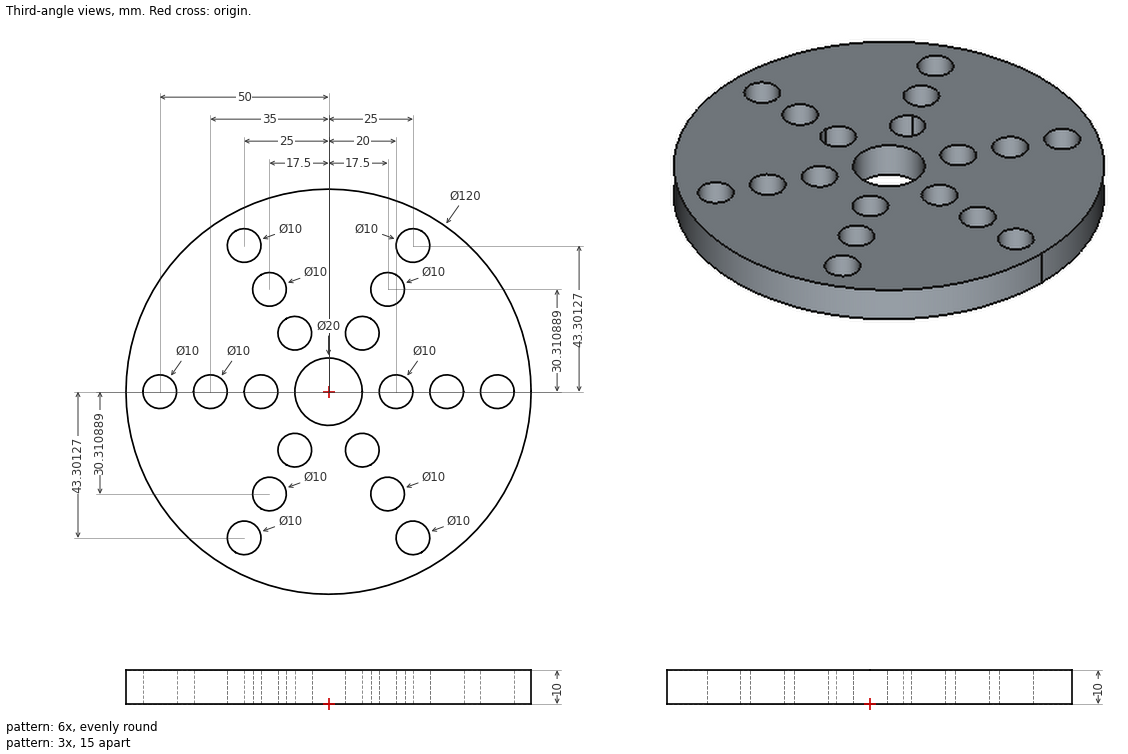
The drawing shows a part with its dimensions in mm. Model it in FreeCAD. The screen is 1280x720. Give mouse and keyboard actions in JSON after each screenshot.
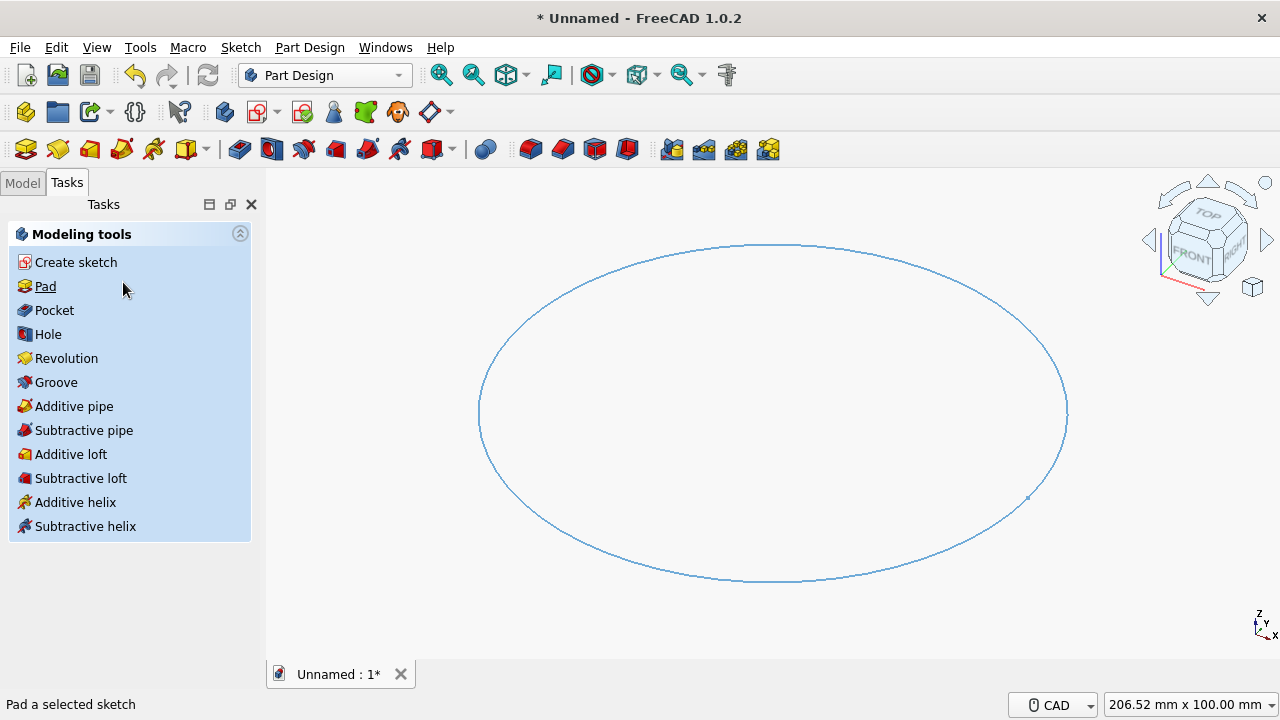
{"action": "left_click", "coordinate": [26, 150]}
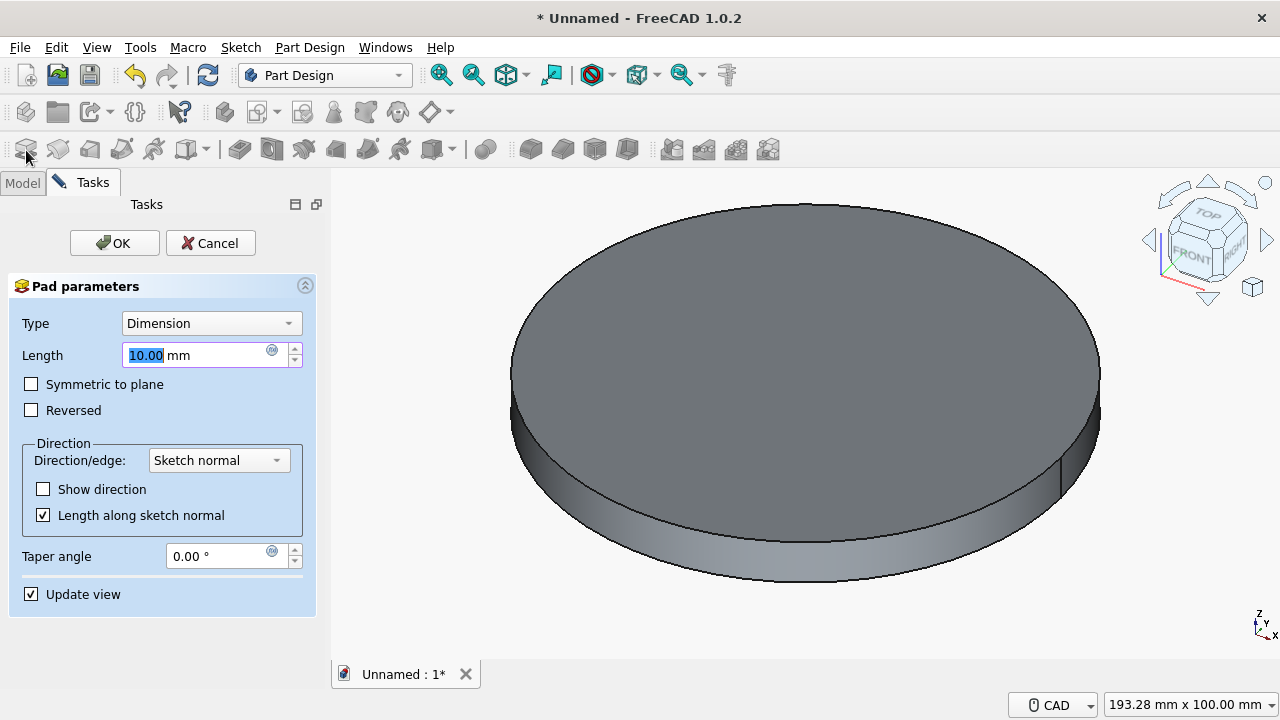
{"action": "type", "text": "10"}
{"action": "key", "text": "Tab"}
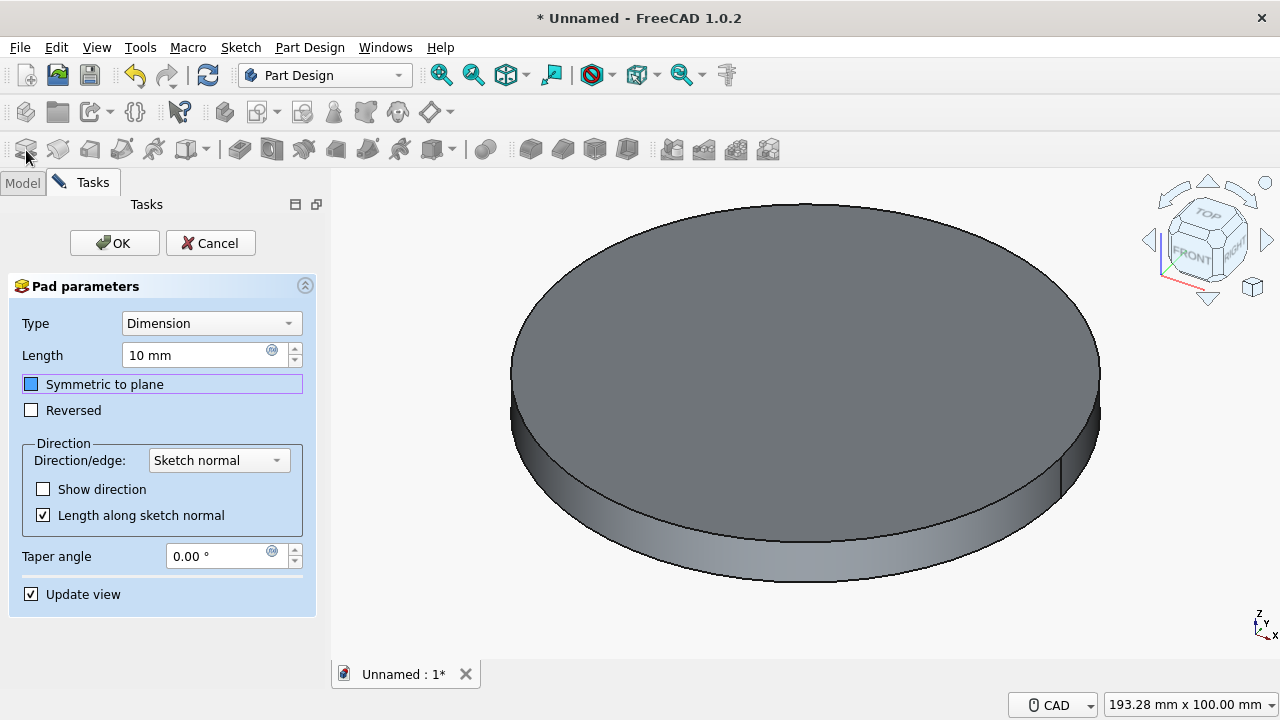
{"action": "left_click", "coordinate": [115, 243]}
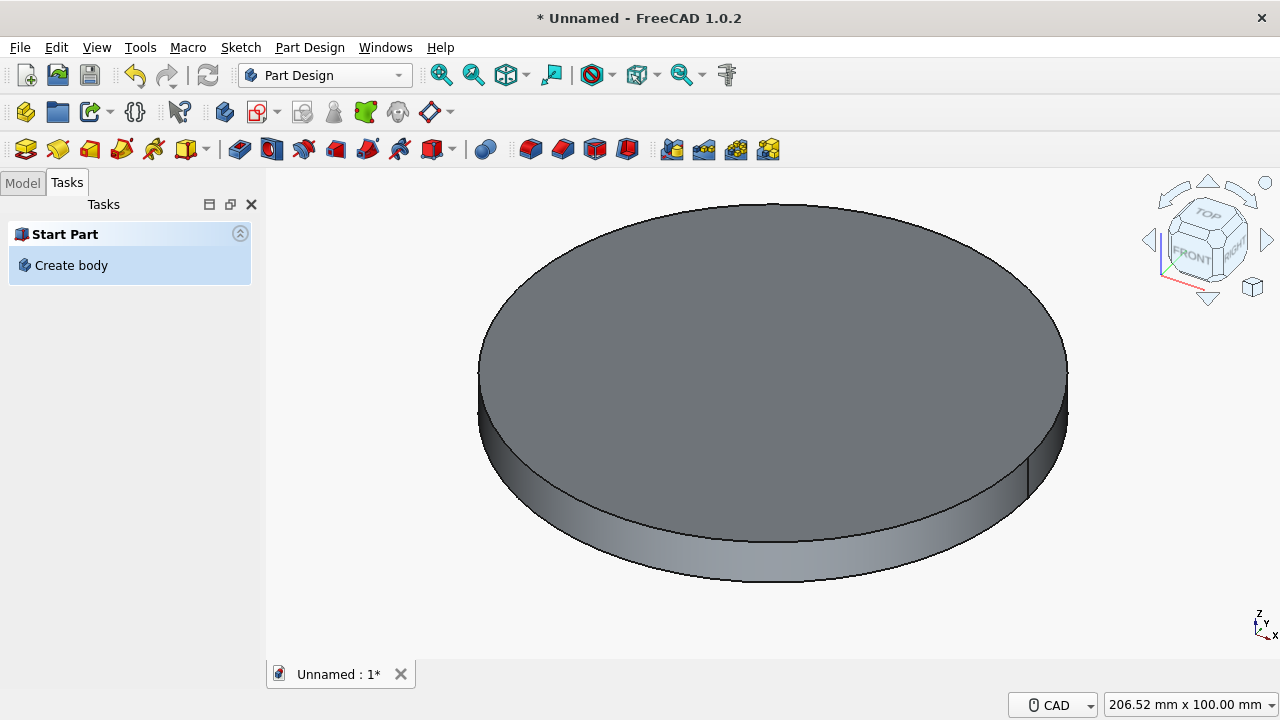
{"action": "left_click", "coordinate": [442, 76]}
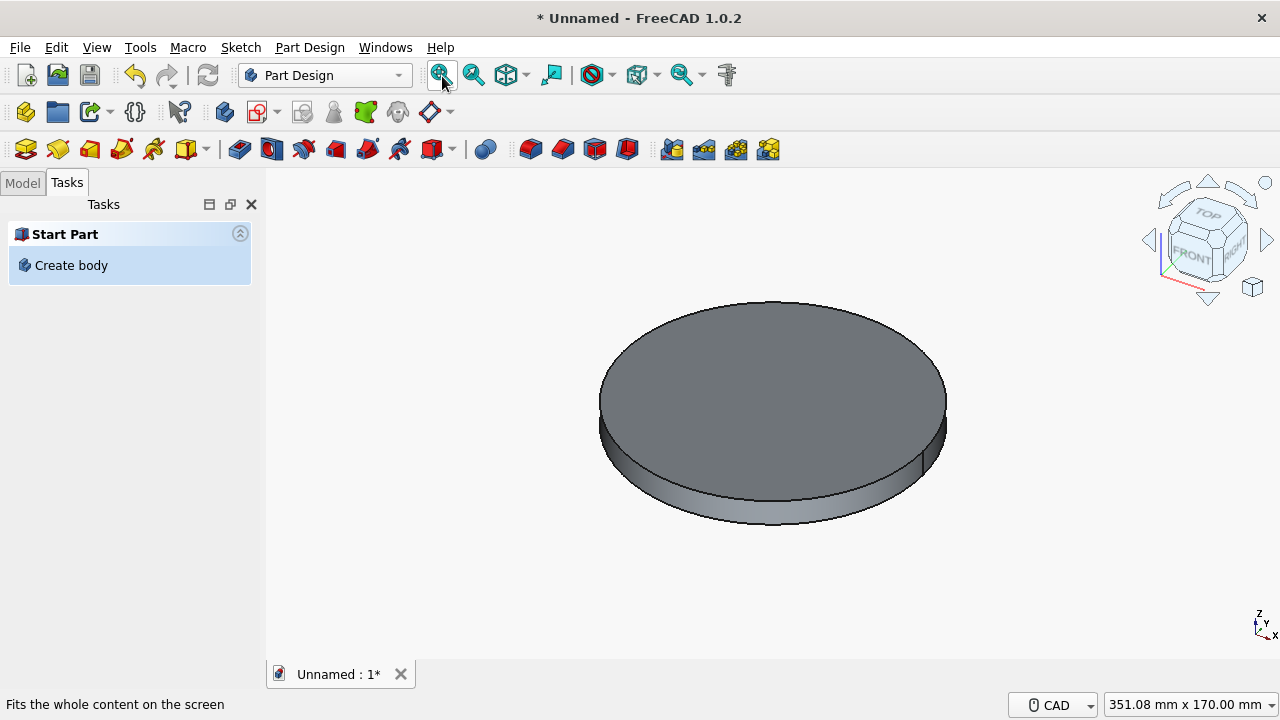
{"action": "left_click", "coordinate": [773, 401]}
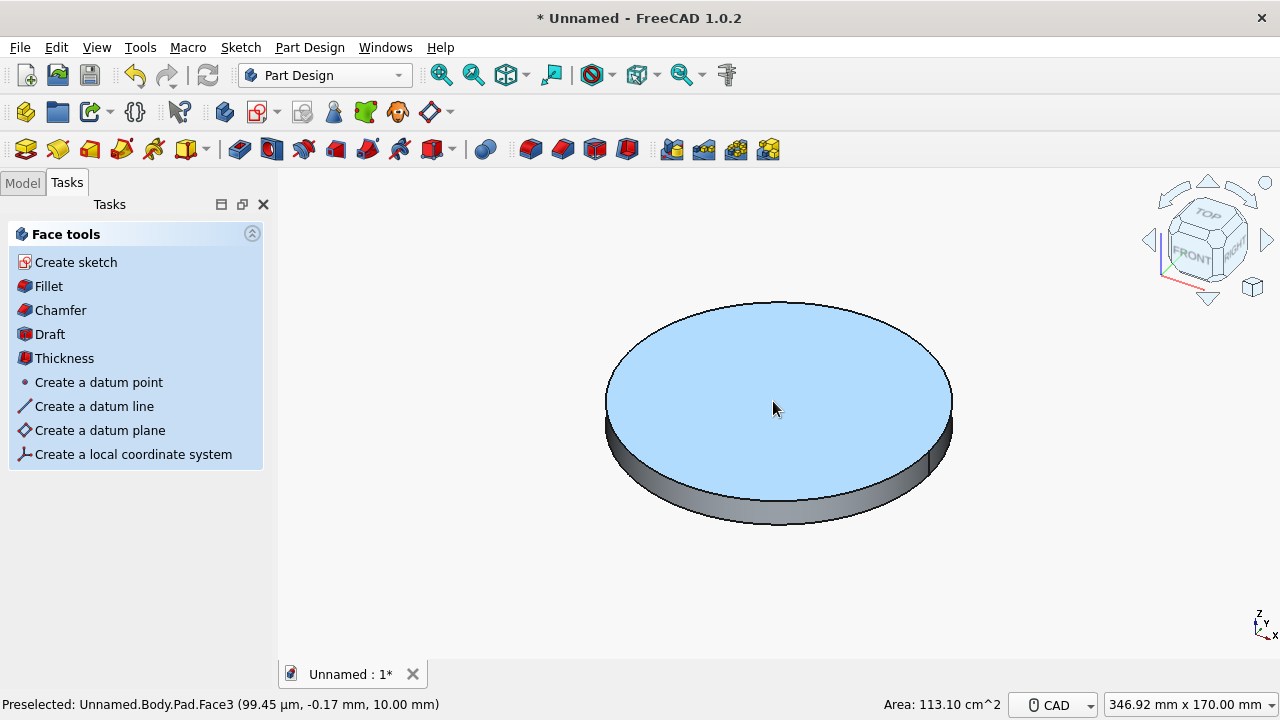
{"action": "left_click", "coordinate": [258, 112]}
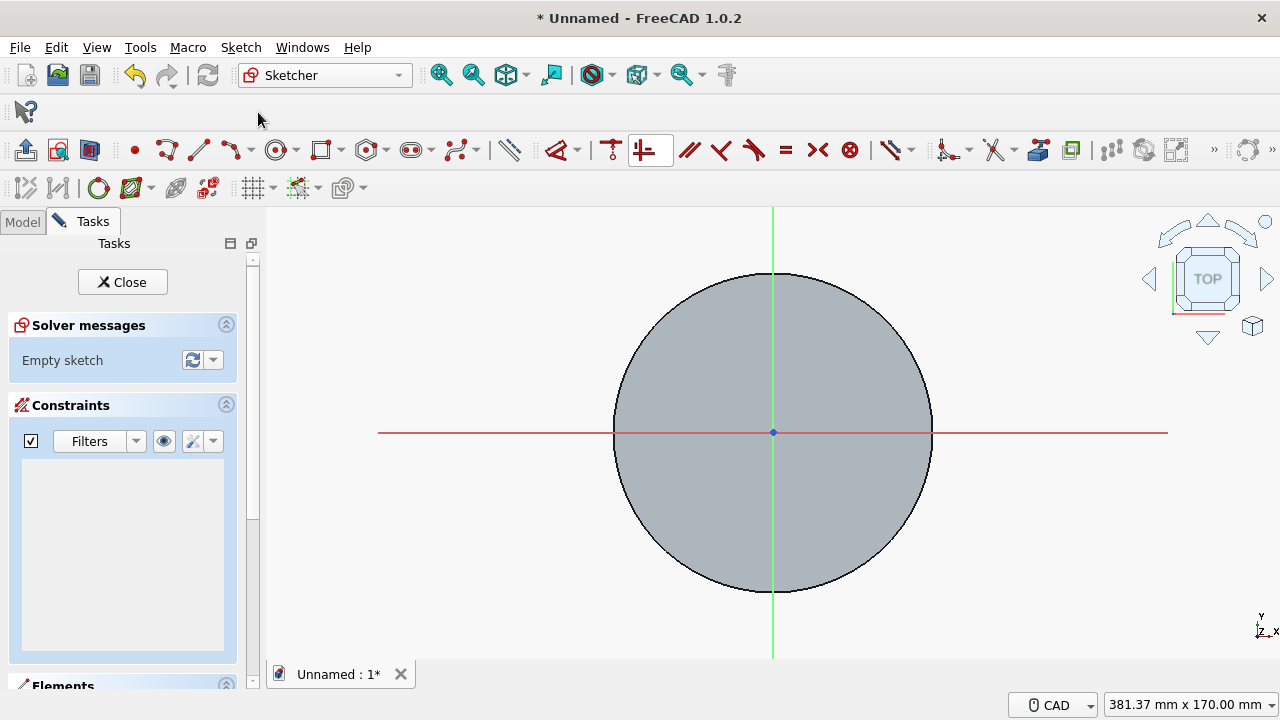
{"action": "scroll", "coordinate": [790, 433], "scroll_direction": "up", "scroll_amount": 8}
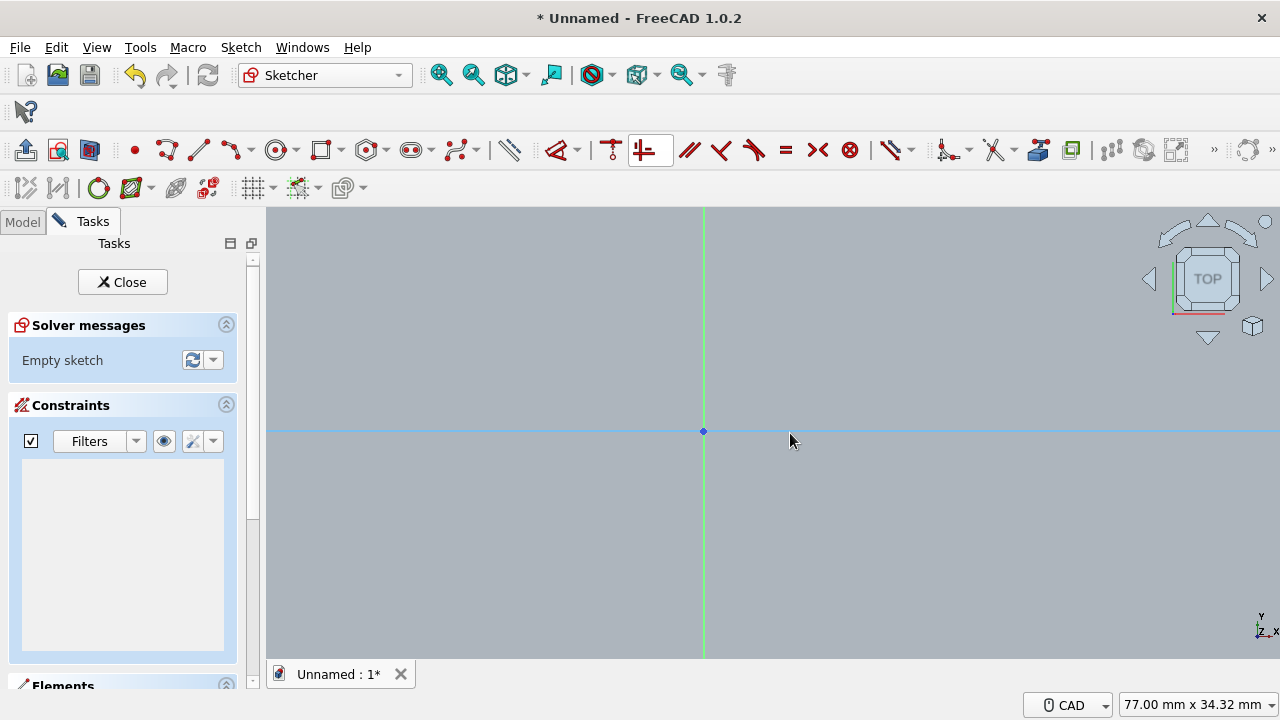
{"action": "left_click", "coordinate": [276, 150]}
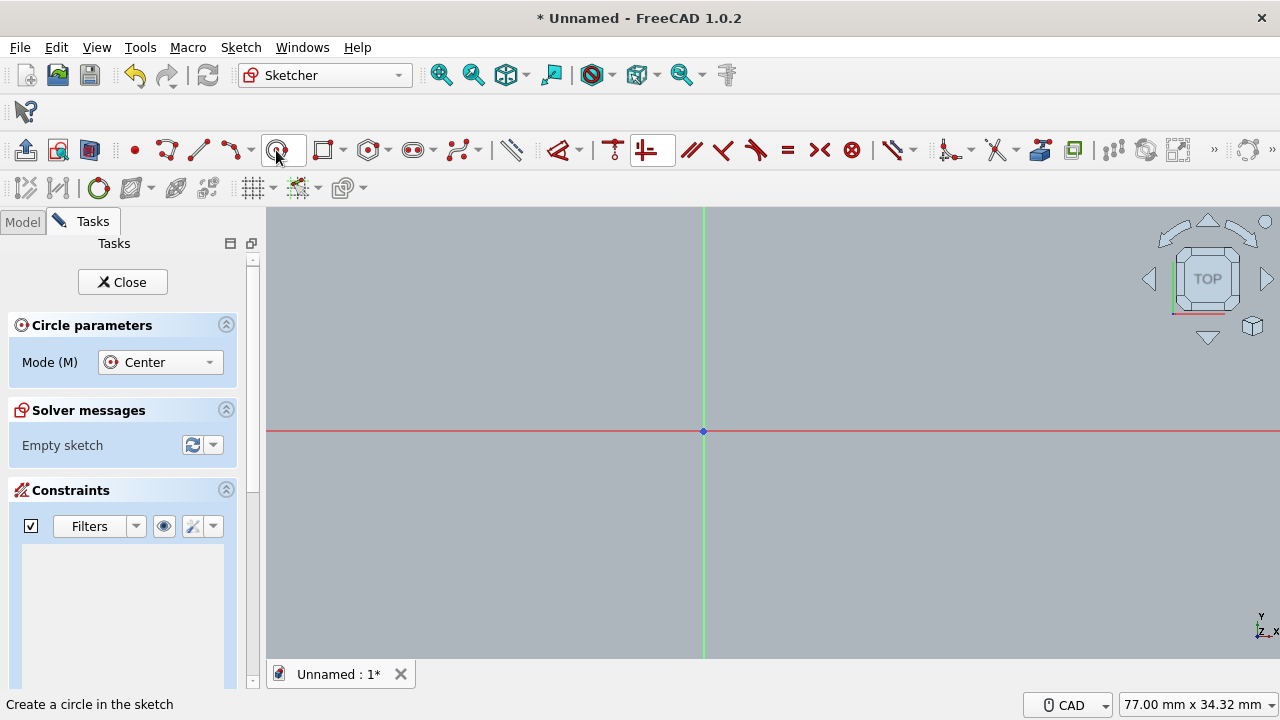
{"action": "left_click", "coordinate": [704, 431]}
{"action": "left_click", "coordinate": [797, 338]}
{"action": "key", "text": "Escape"}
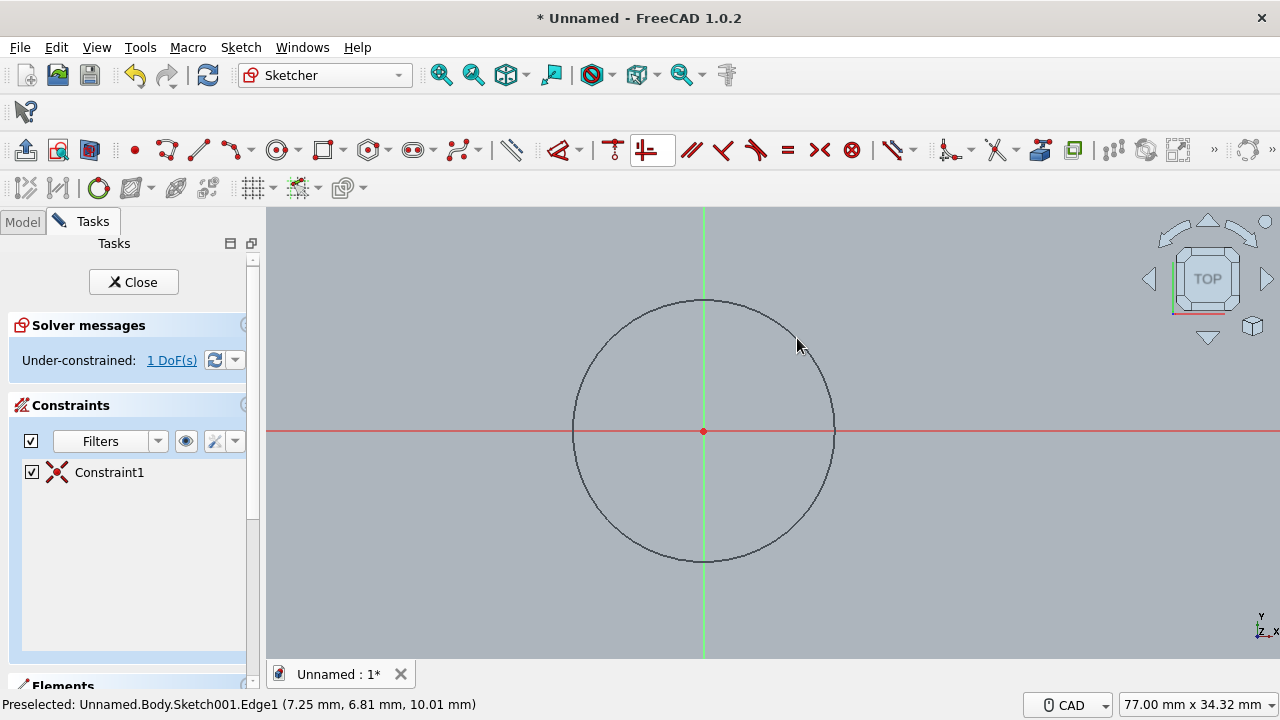
{"action": "left_click", "coordinate": [558, 150]}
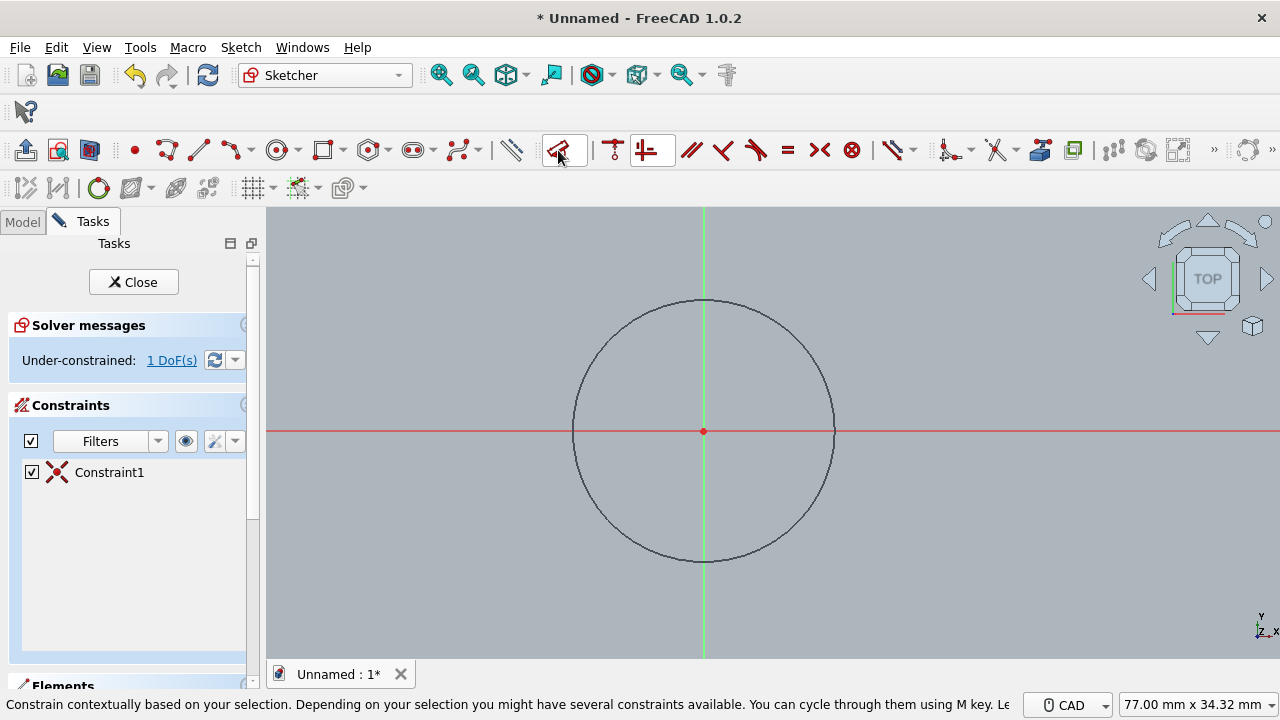
{"action": "left_click", "coordinate": [796, 338]}
{"action": "left_click", "coordinate": [819, 315]}